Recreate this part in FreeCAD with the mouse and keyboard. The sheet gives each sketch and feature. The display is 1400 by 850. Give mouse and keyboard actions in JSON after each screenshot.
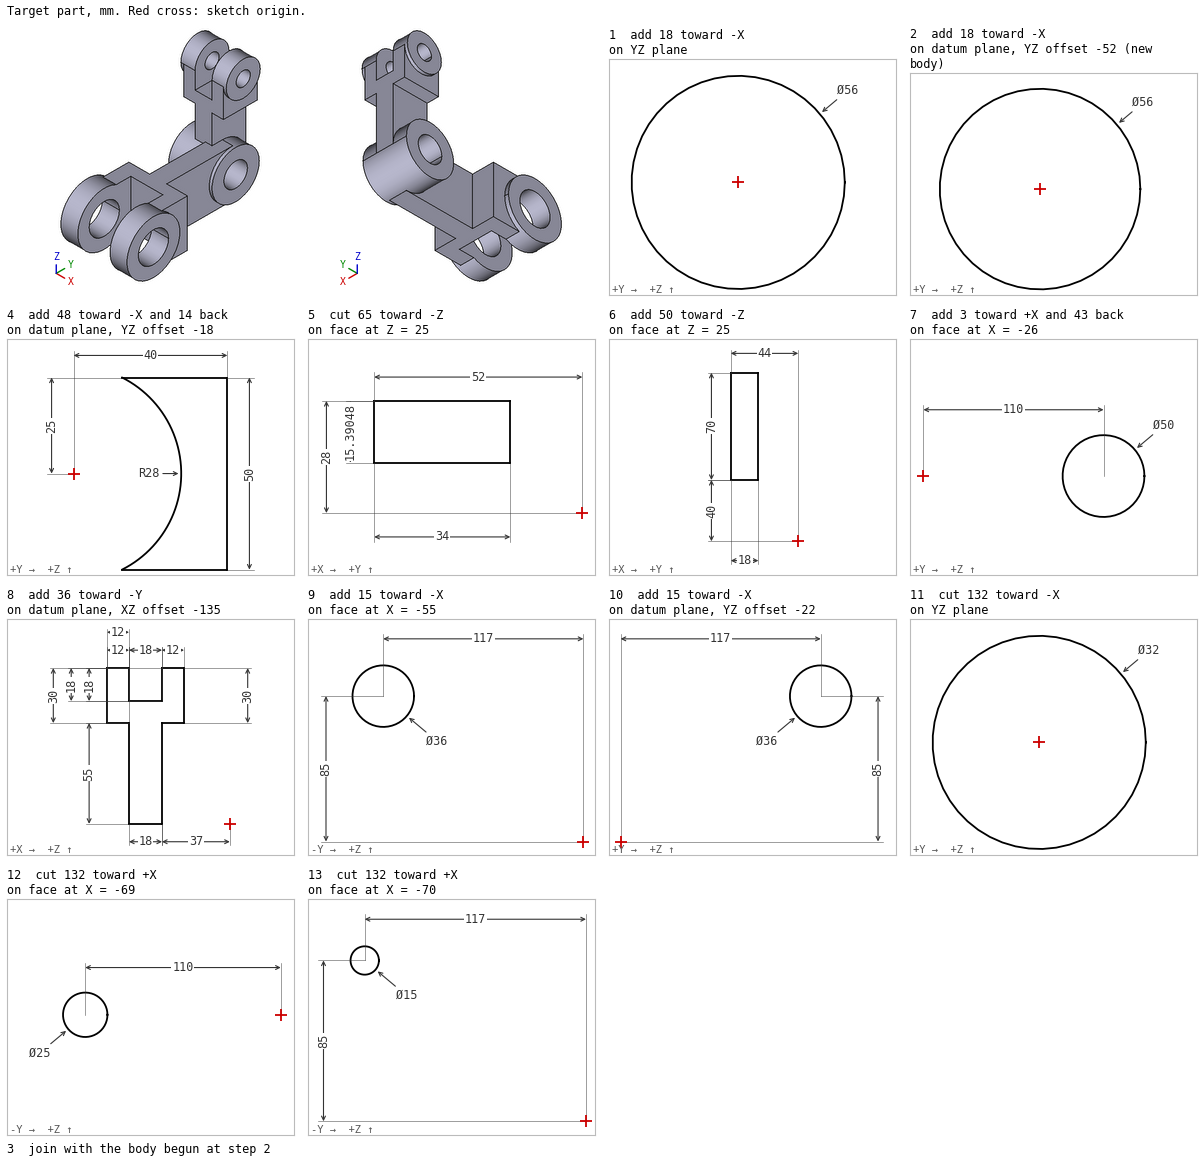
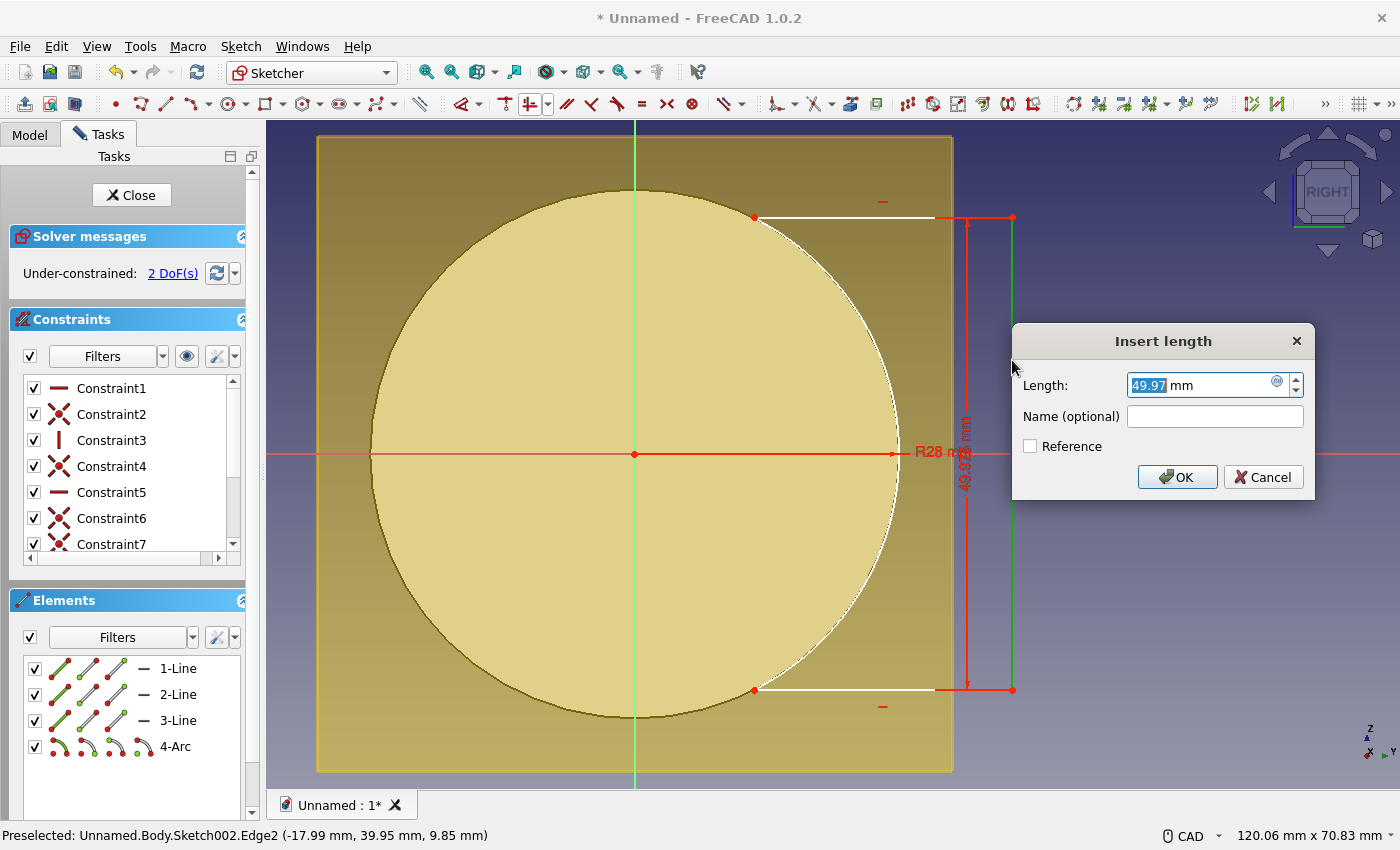
{"action": "type", "text": "50"}
{"action": "key", "text": "Return"}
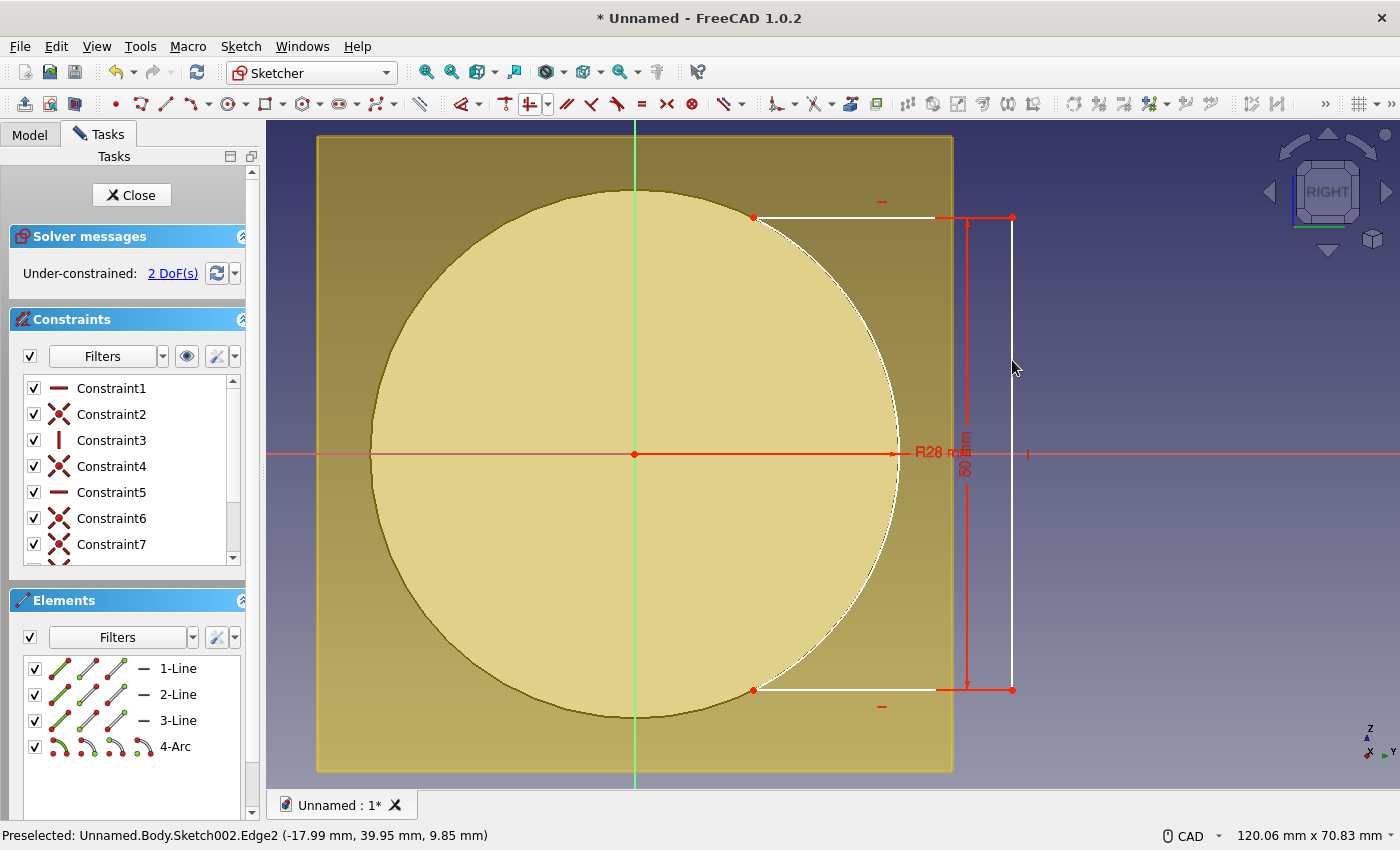
{"action": "left_click", "coordinate": [754, 218]}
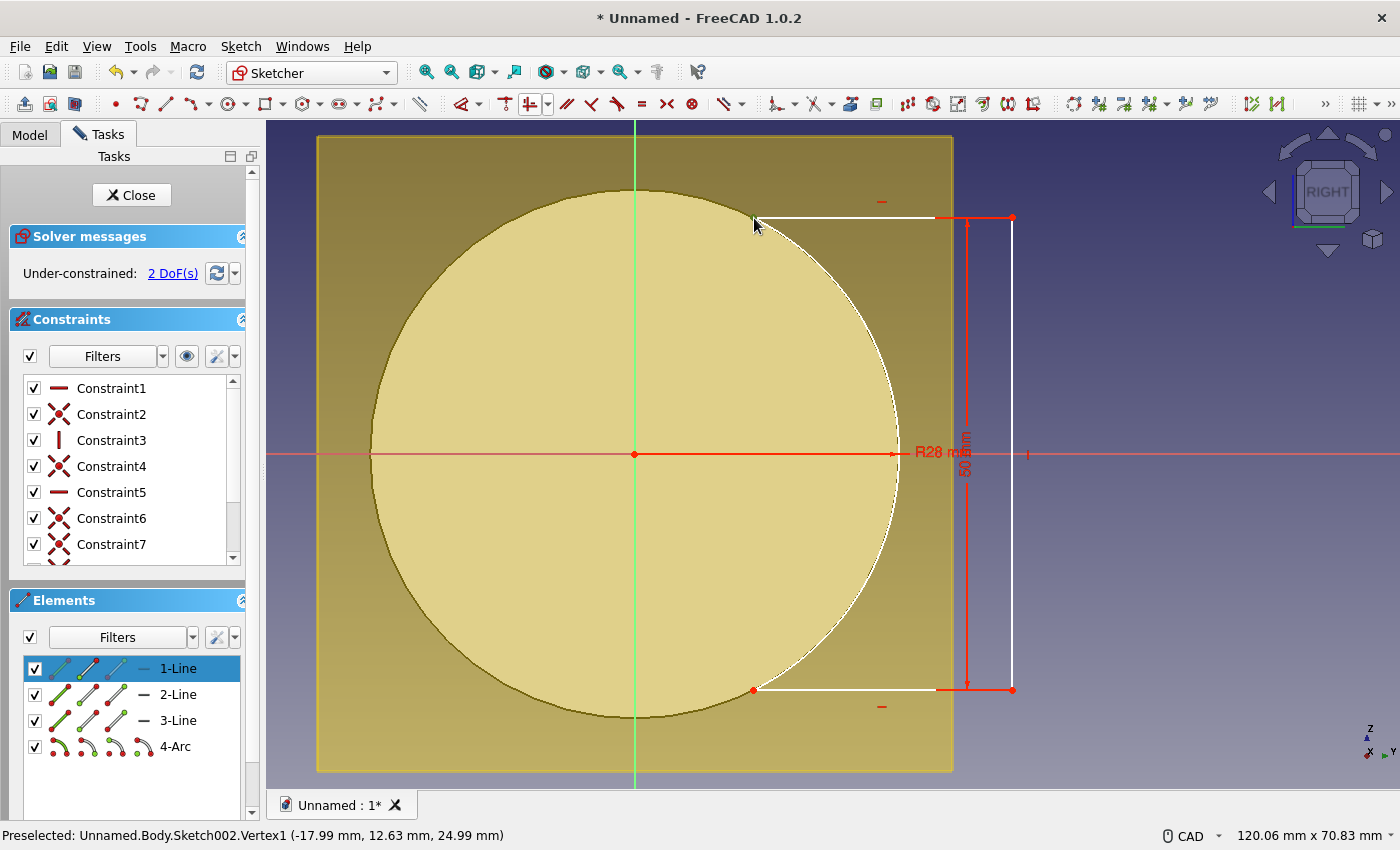
{"action": "key", "text": "i"}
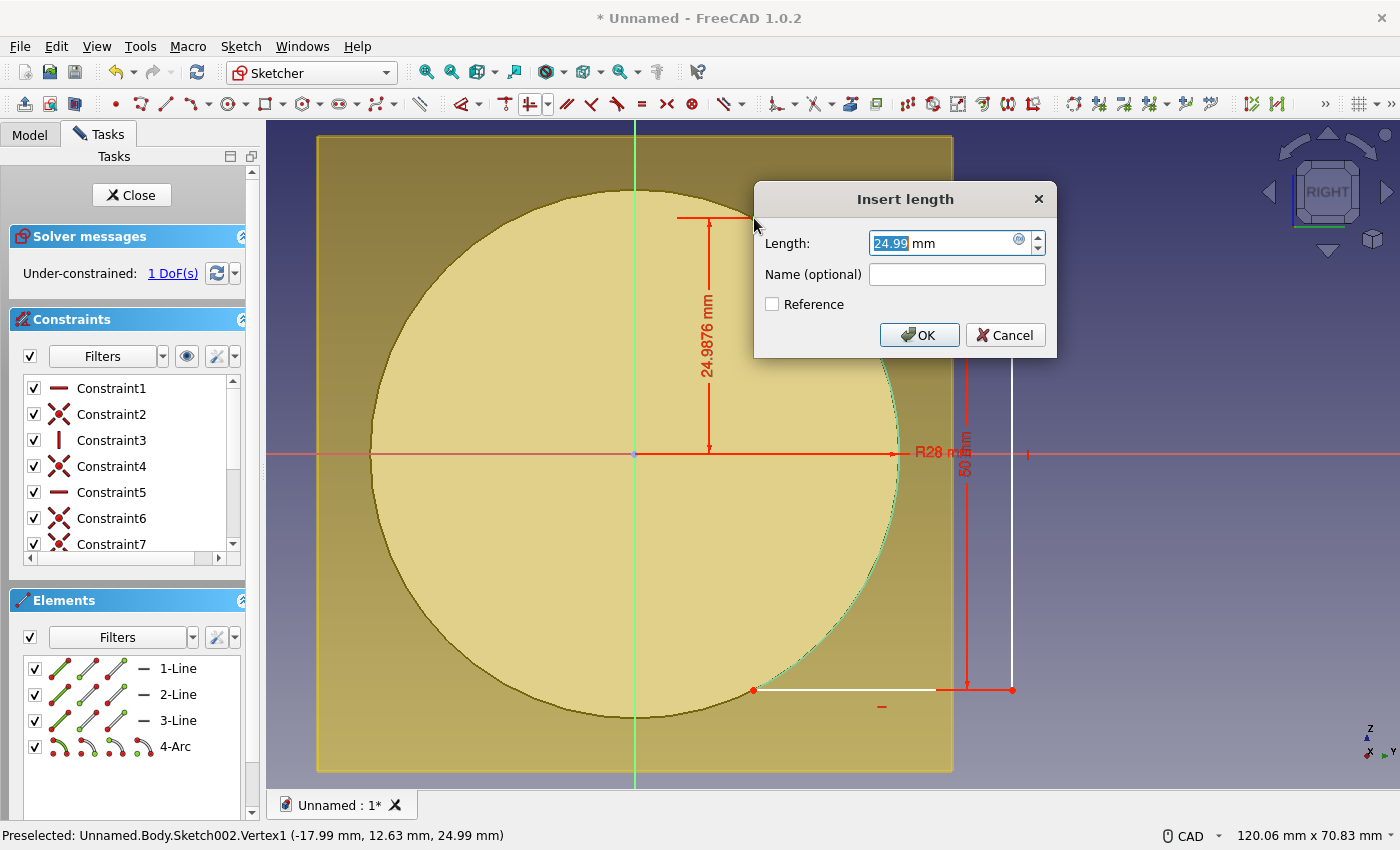
{"action": "type", "text": "25"}
{"action": "key", "text": "Return"}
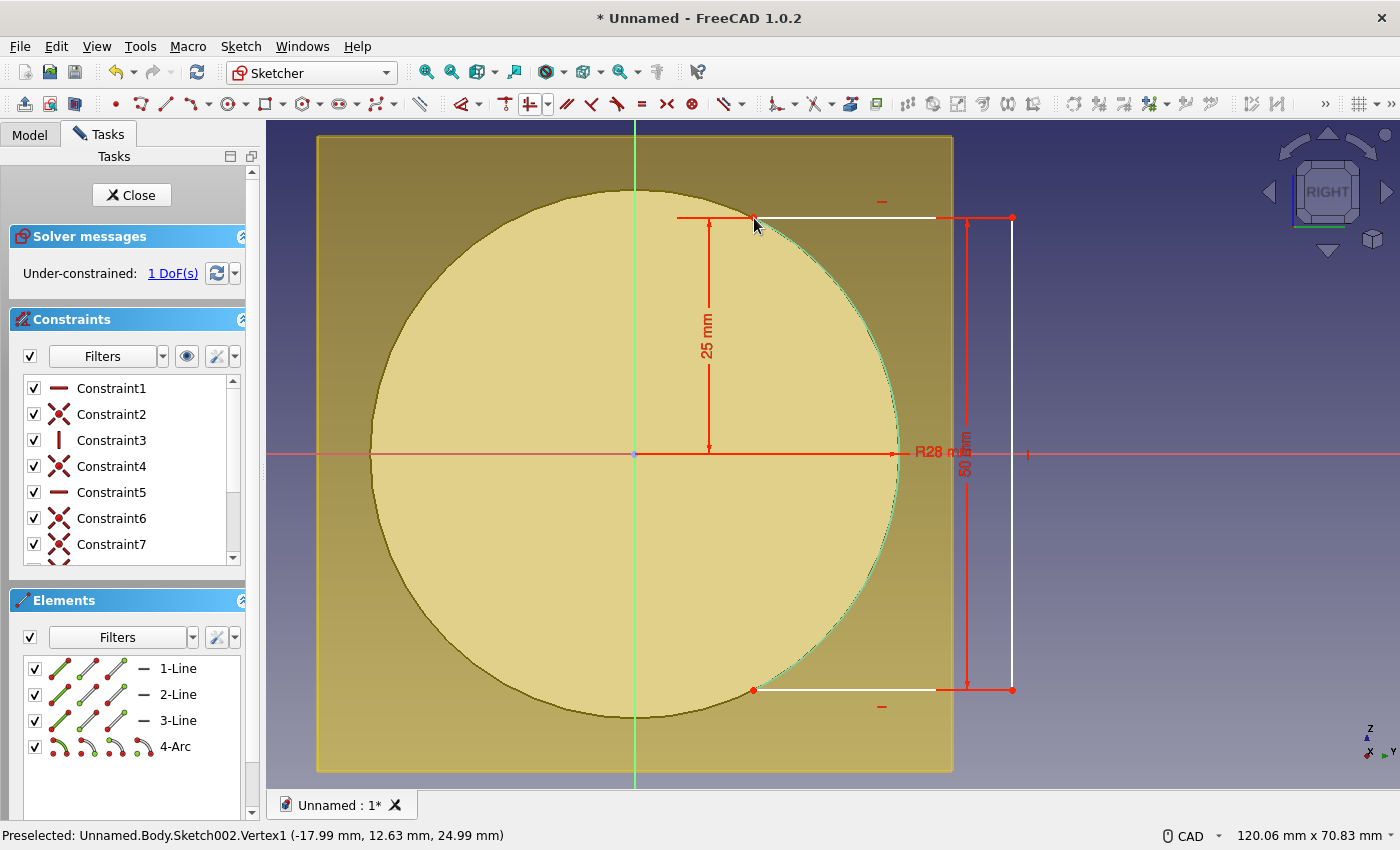
{"action": "left_click", "coordinate": [1012, 218]}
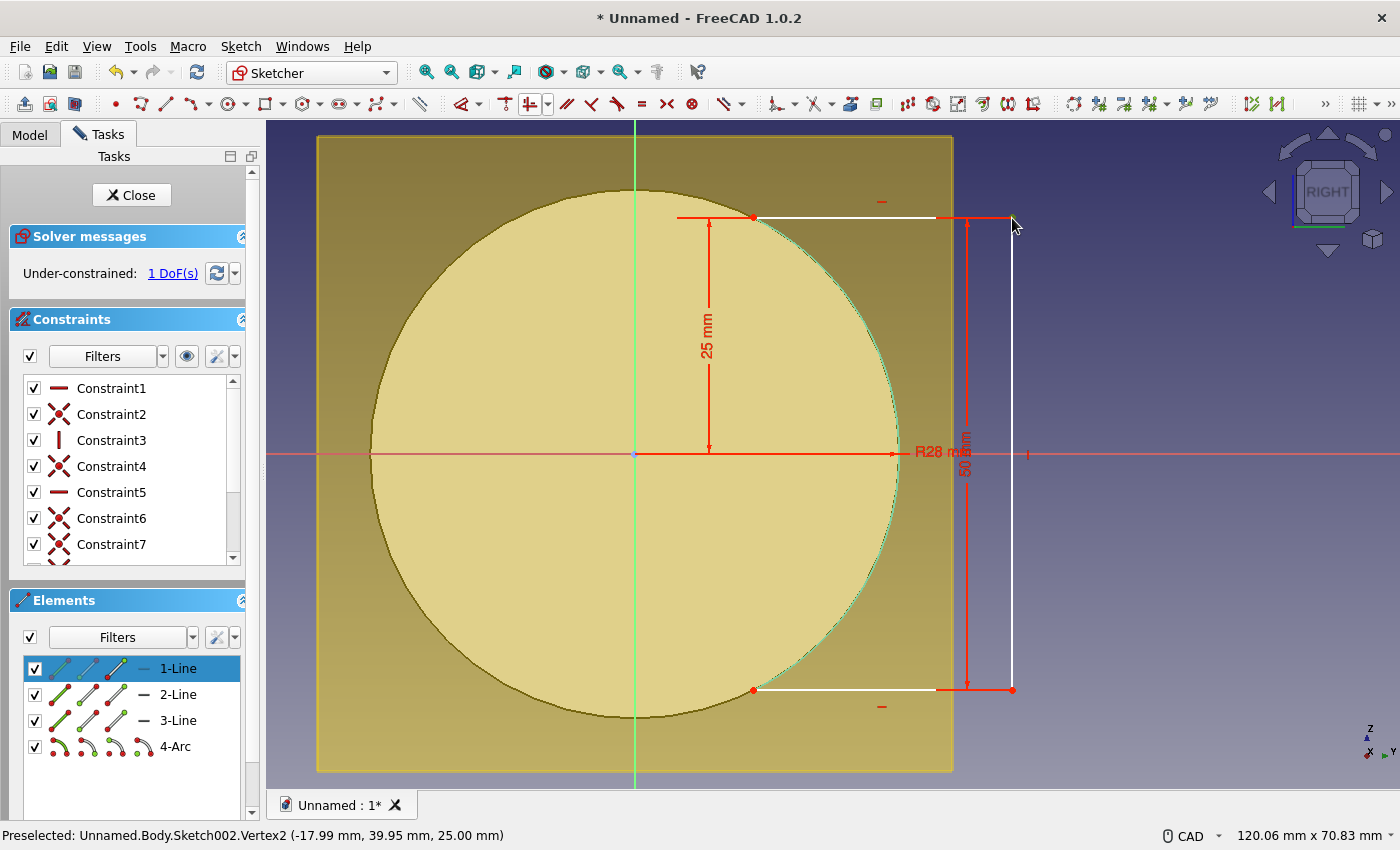
{"action": "key", "text": "l"}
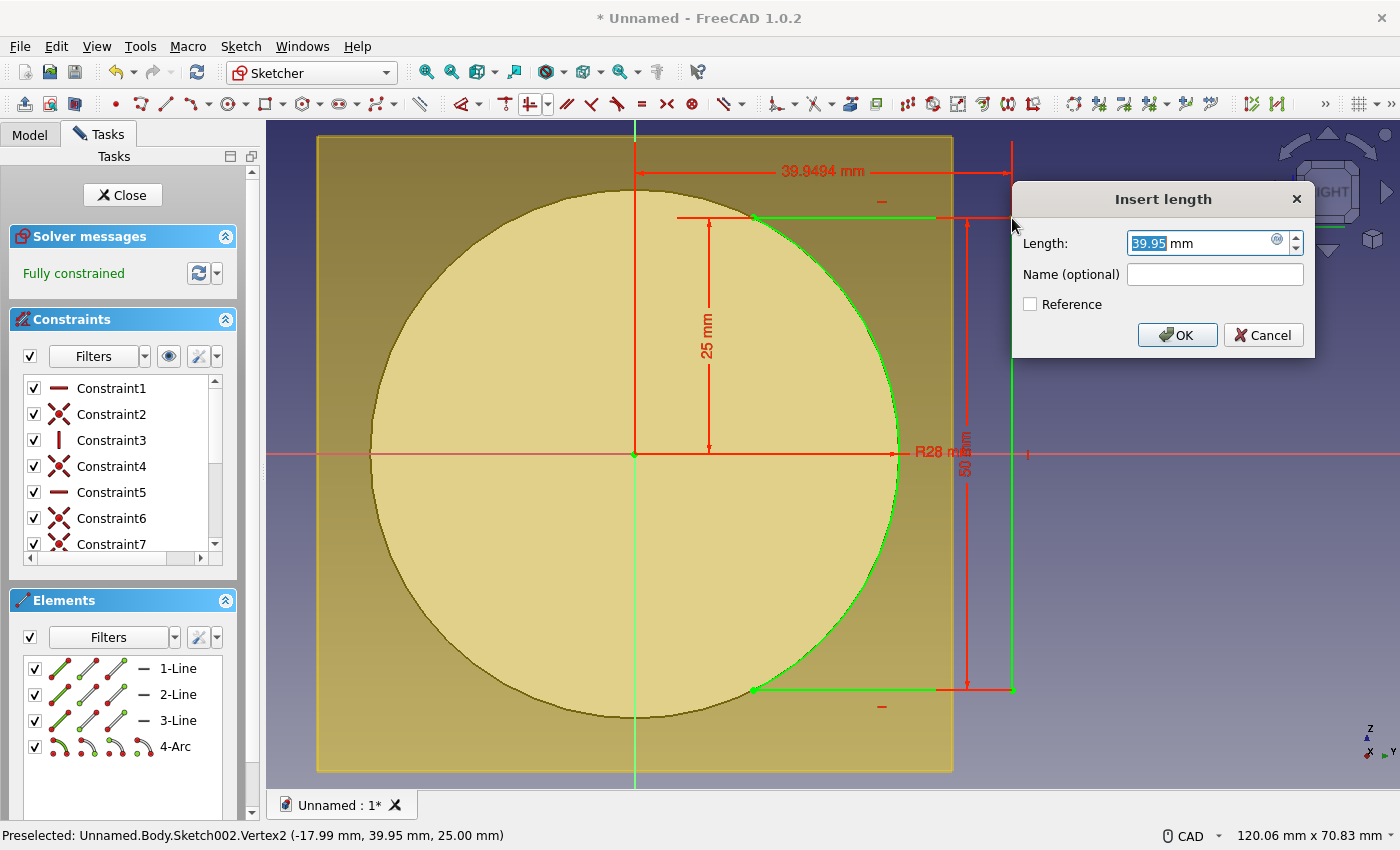
{"action": "type", "text": "40"}
{"action": "key", "text": "Return"}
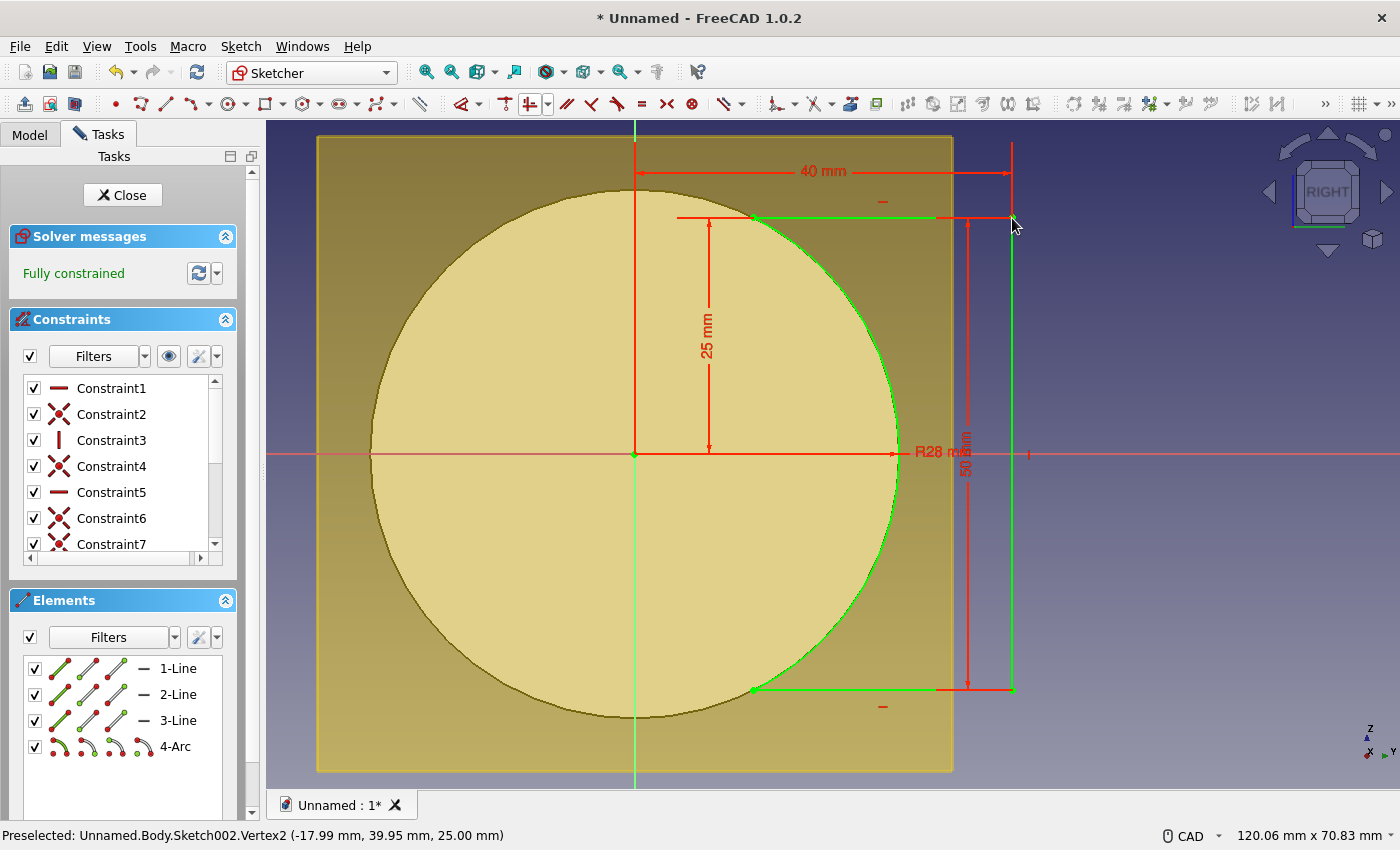
{"action": "left_click", "coordinate": [123, 195]}